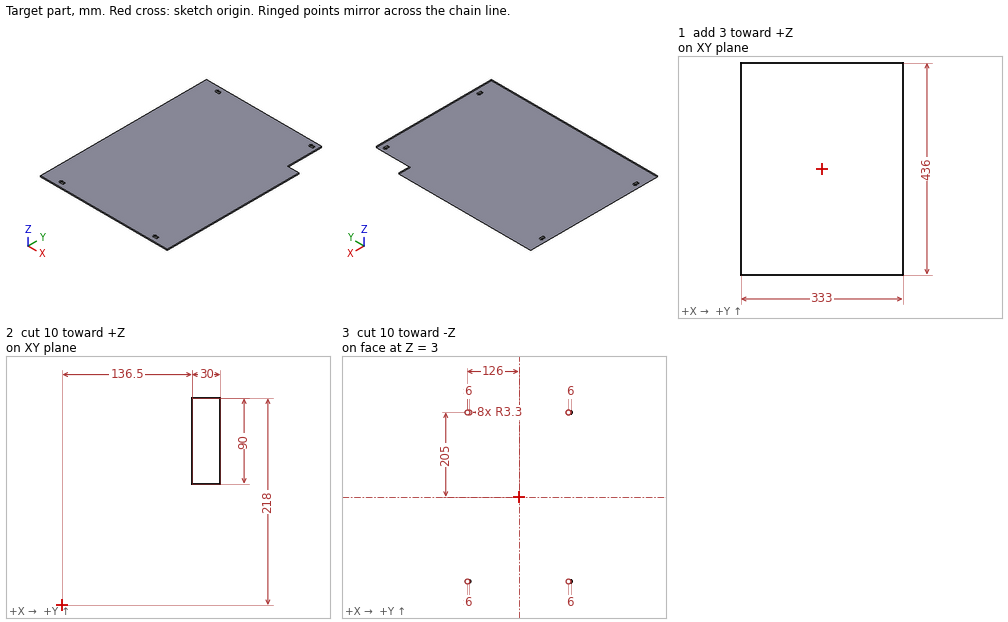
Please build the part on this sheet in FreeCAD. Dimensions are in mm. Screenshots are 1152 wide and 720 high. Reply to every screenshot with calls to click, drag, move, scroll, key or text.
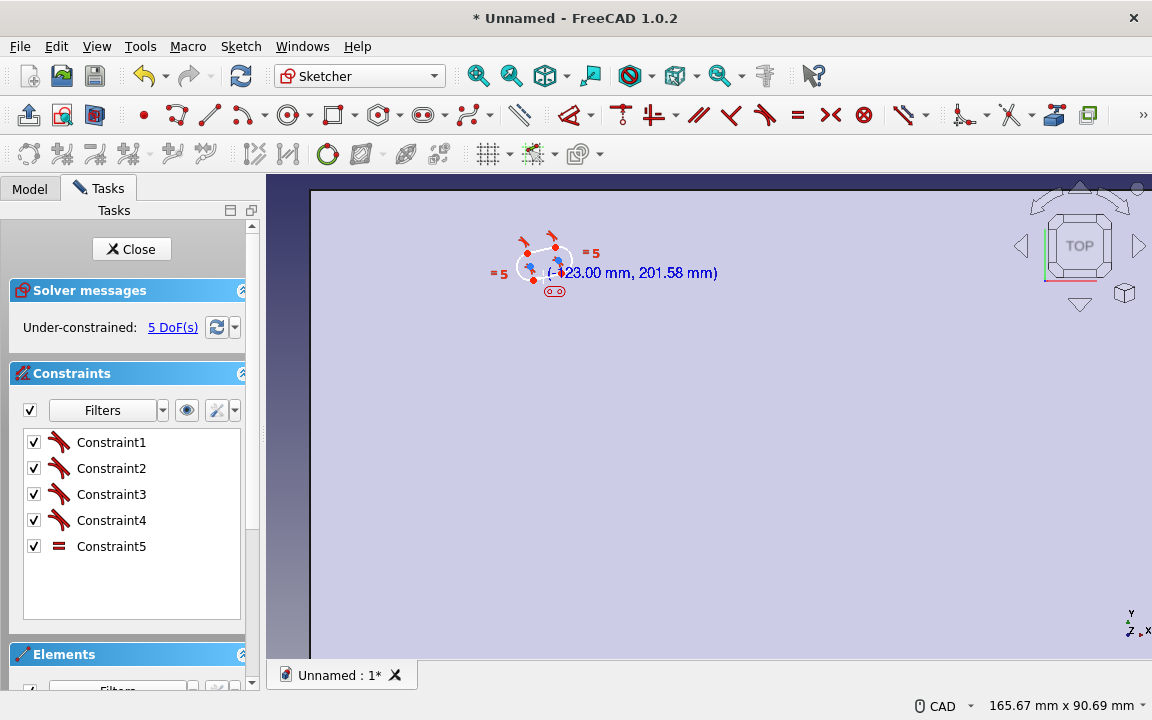
scroll(553, 269, down, 10)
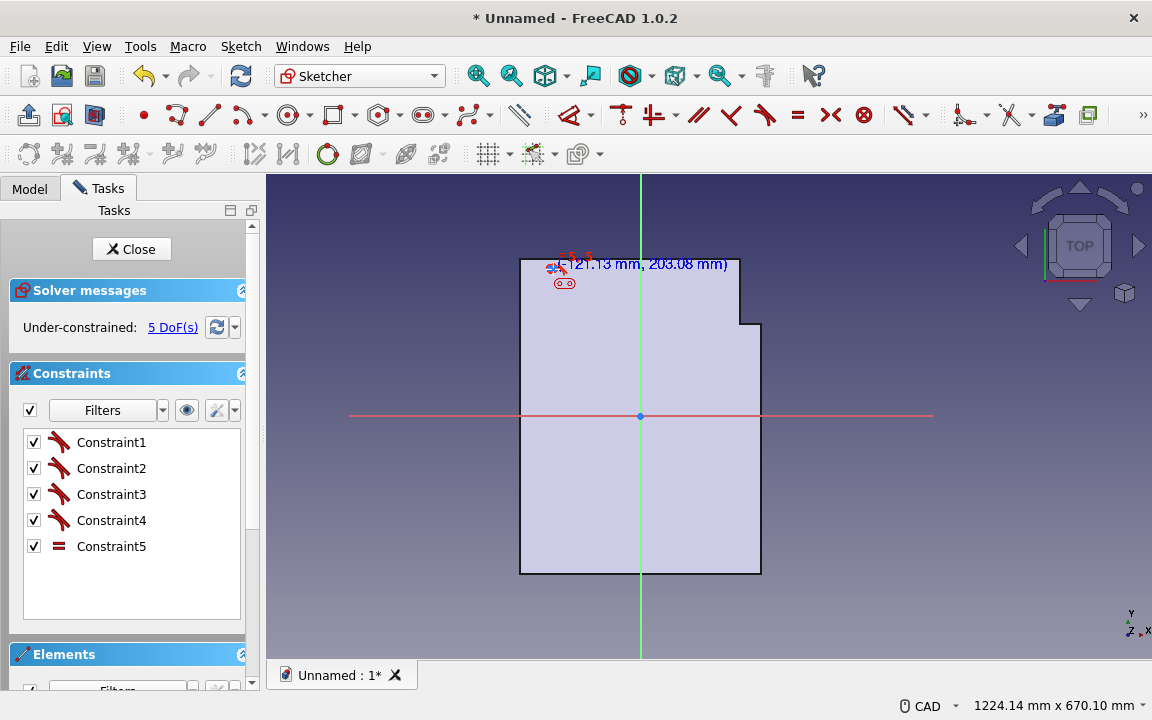
scroll(728, 268, up, 12)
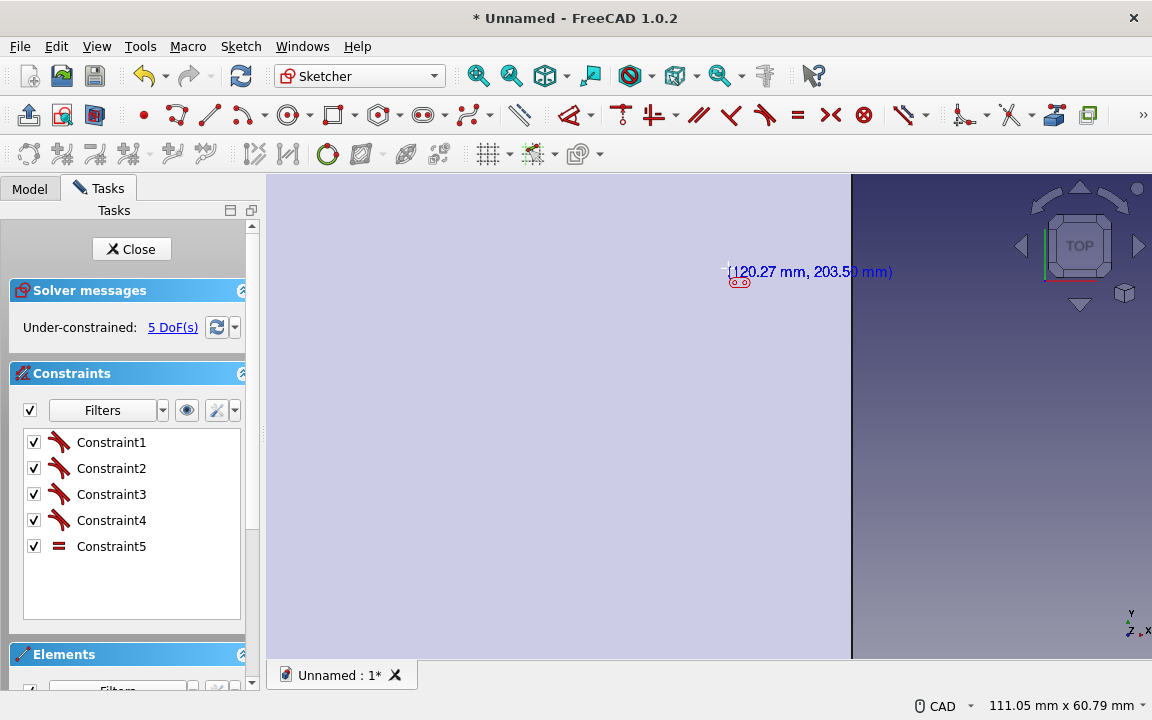
scroll(728, 268, down, 12)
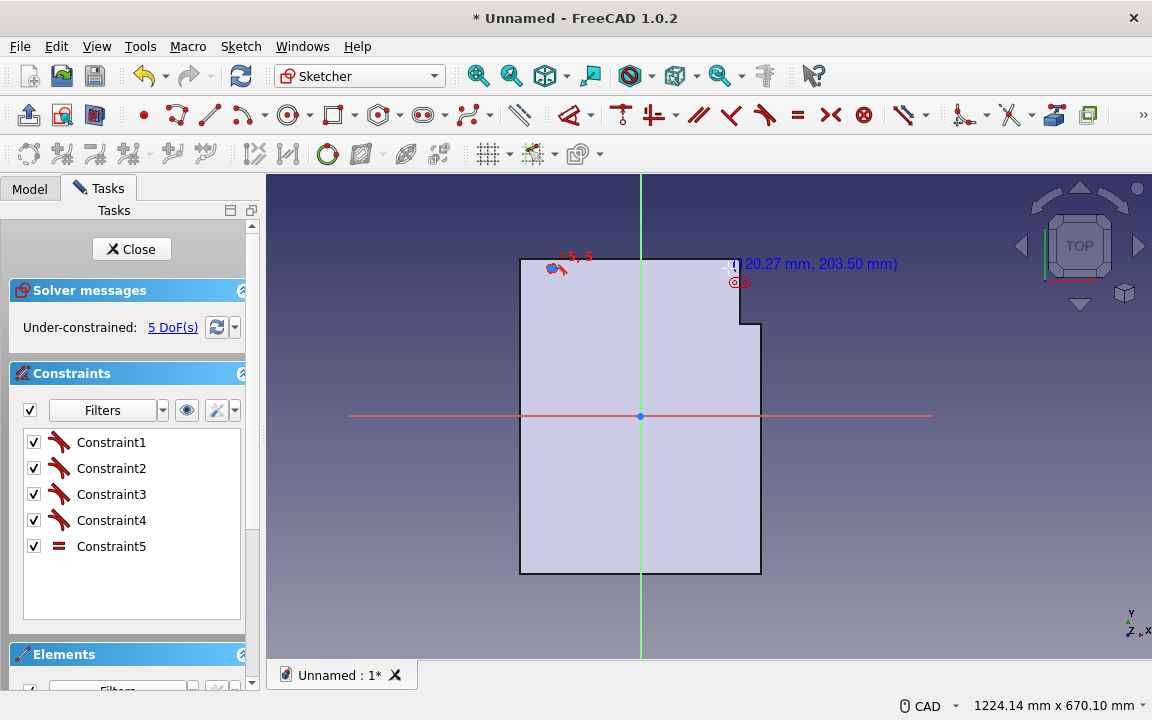
click(728, 268)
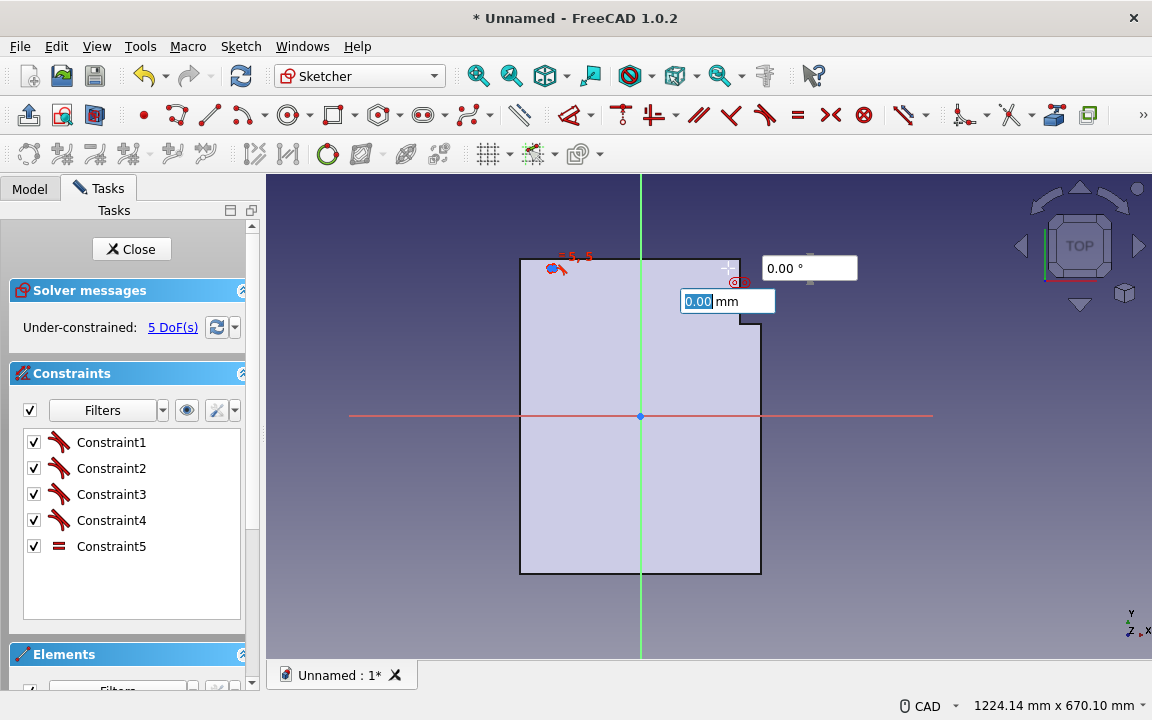
scroll(732, 268, up, 7)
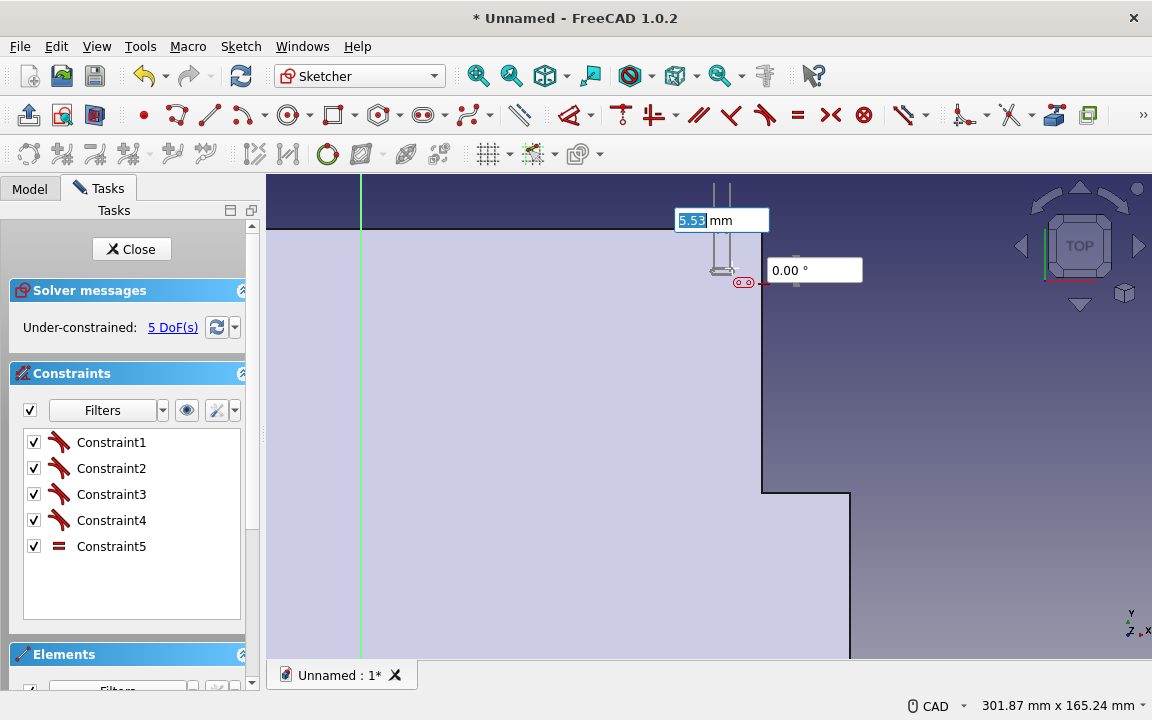
click(731, 267)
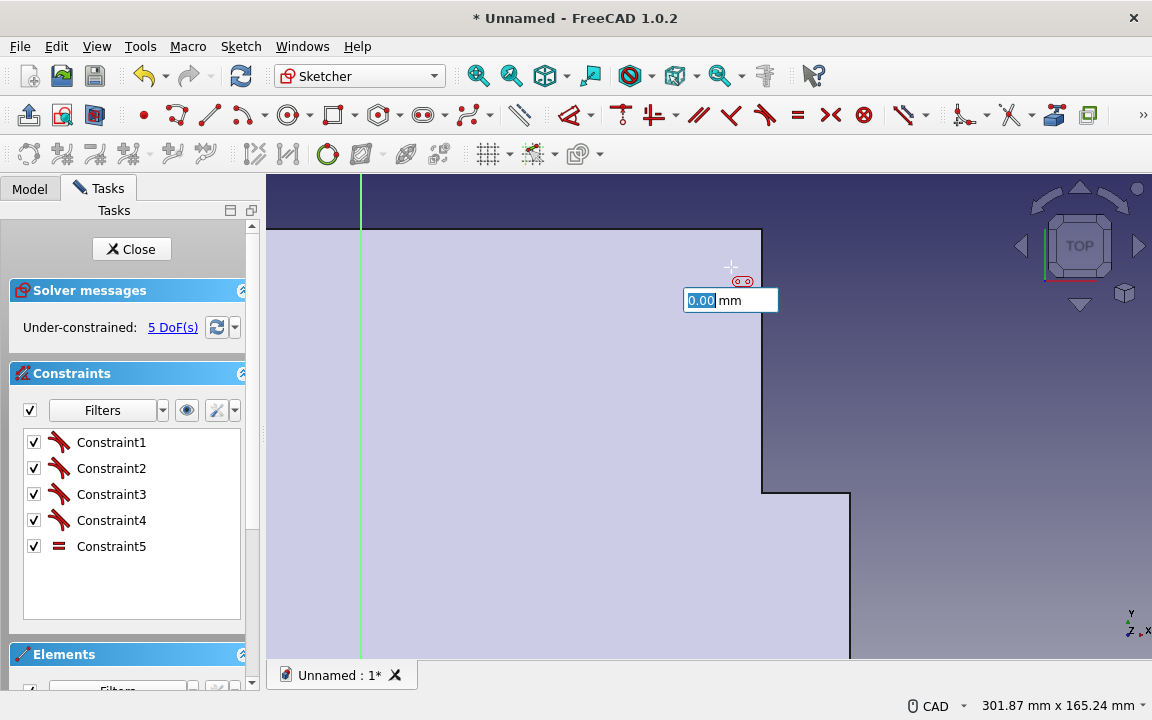
scroll(722, 257, up, 3)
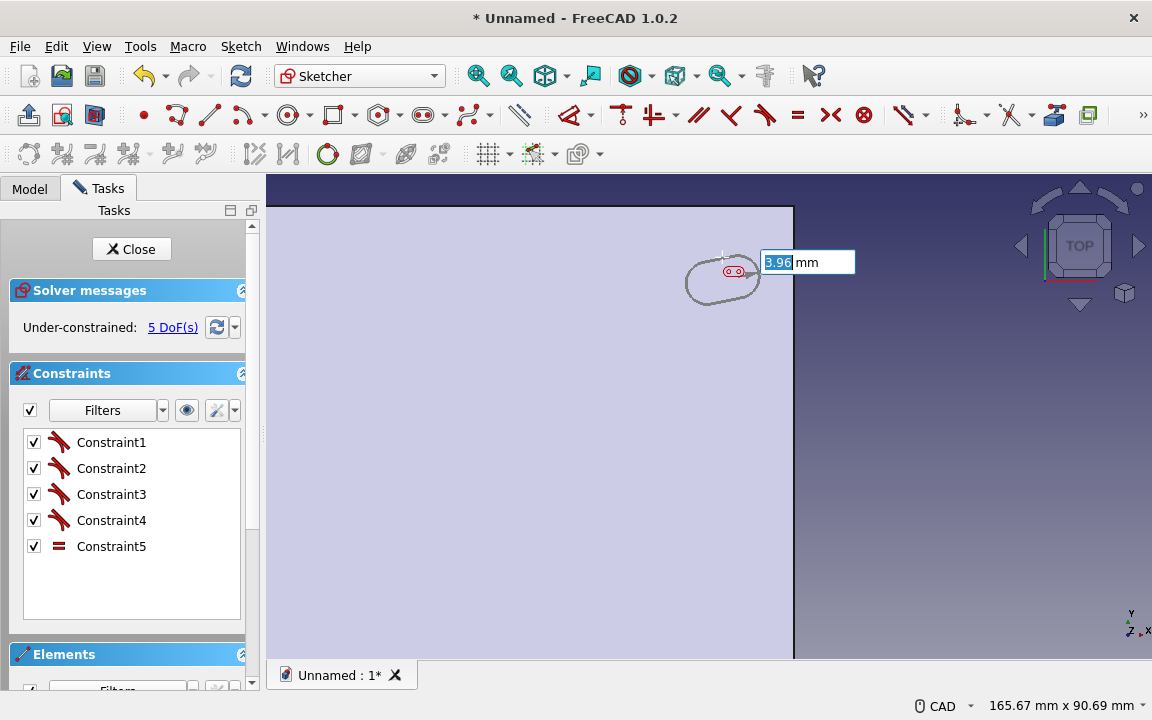
click(722, 258)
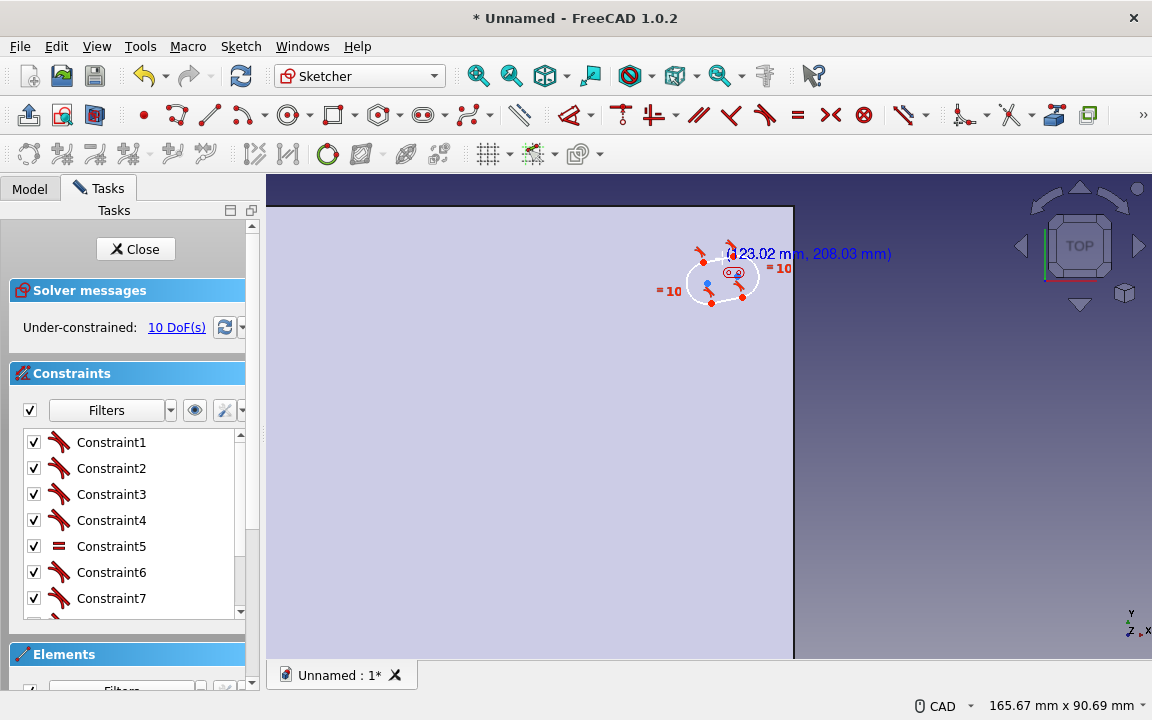
scroll(731, 267, down, 10)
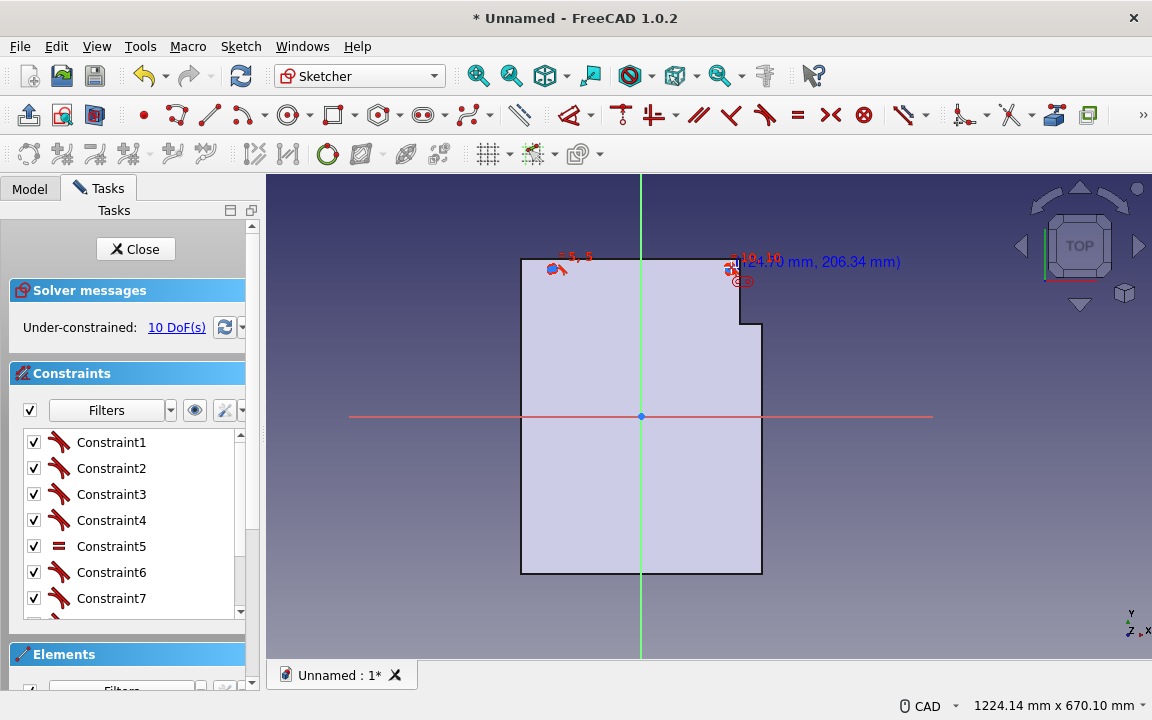
scroll(728, 565, up, 12)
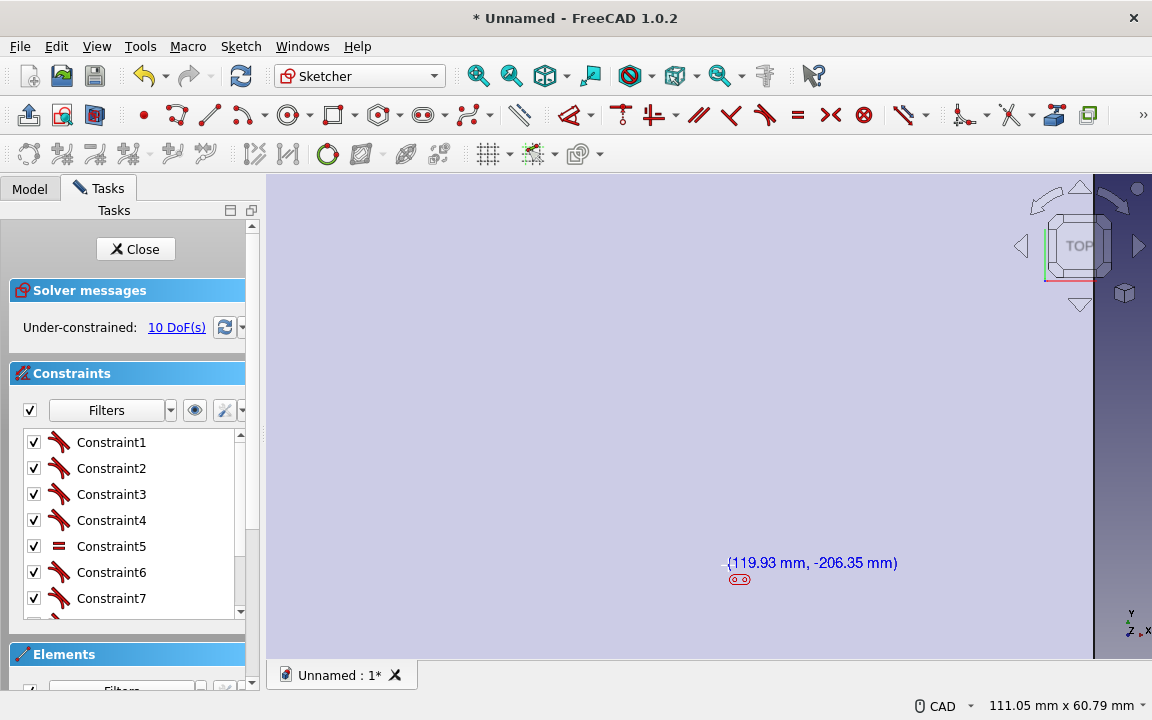
scroll(728, 566, down, 12)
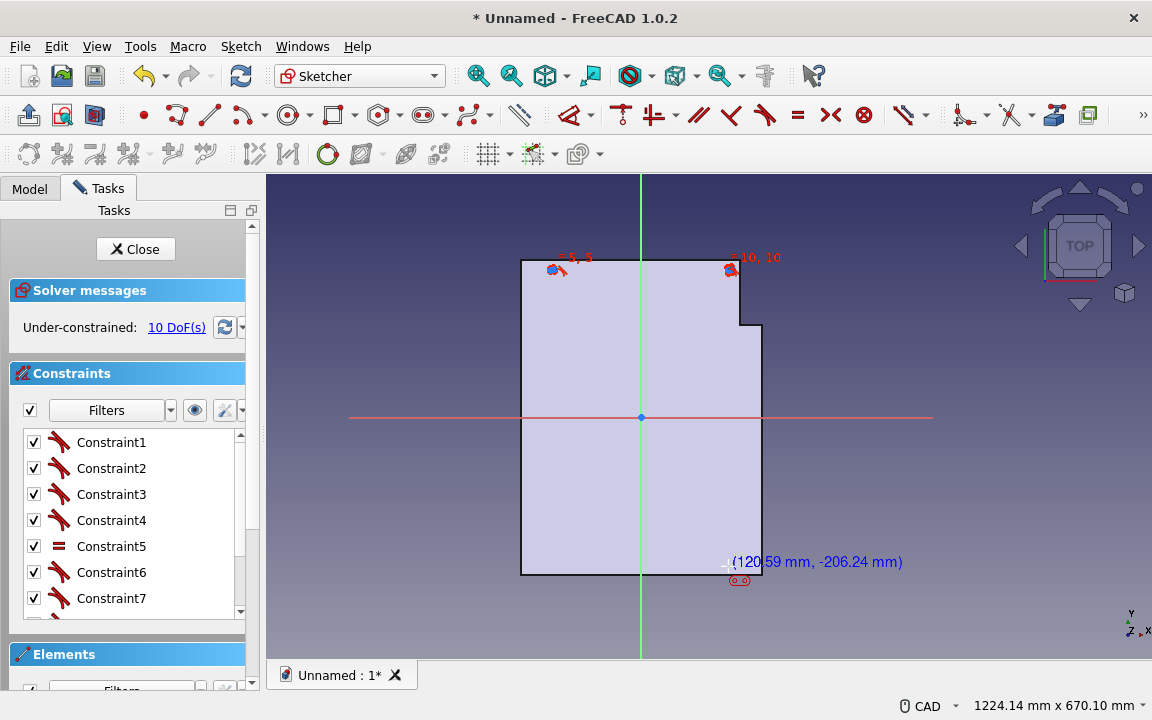
click(728, 566)